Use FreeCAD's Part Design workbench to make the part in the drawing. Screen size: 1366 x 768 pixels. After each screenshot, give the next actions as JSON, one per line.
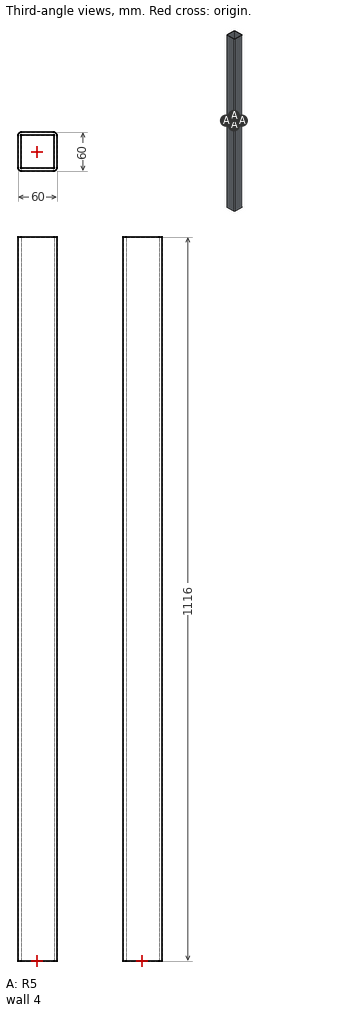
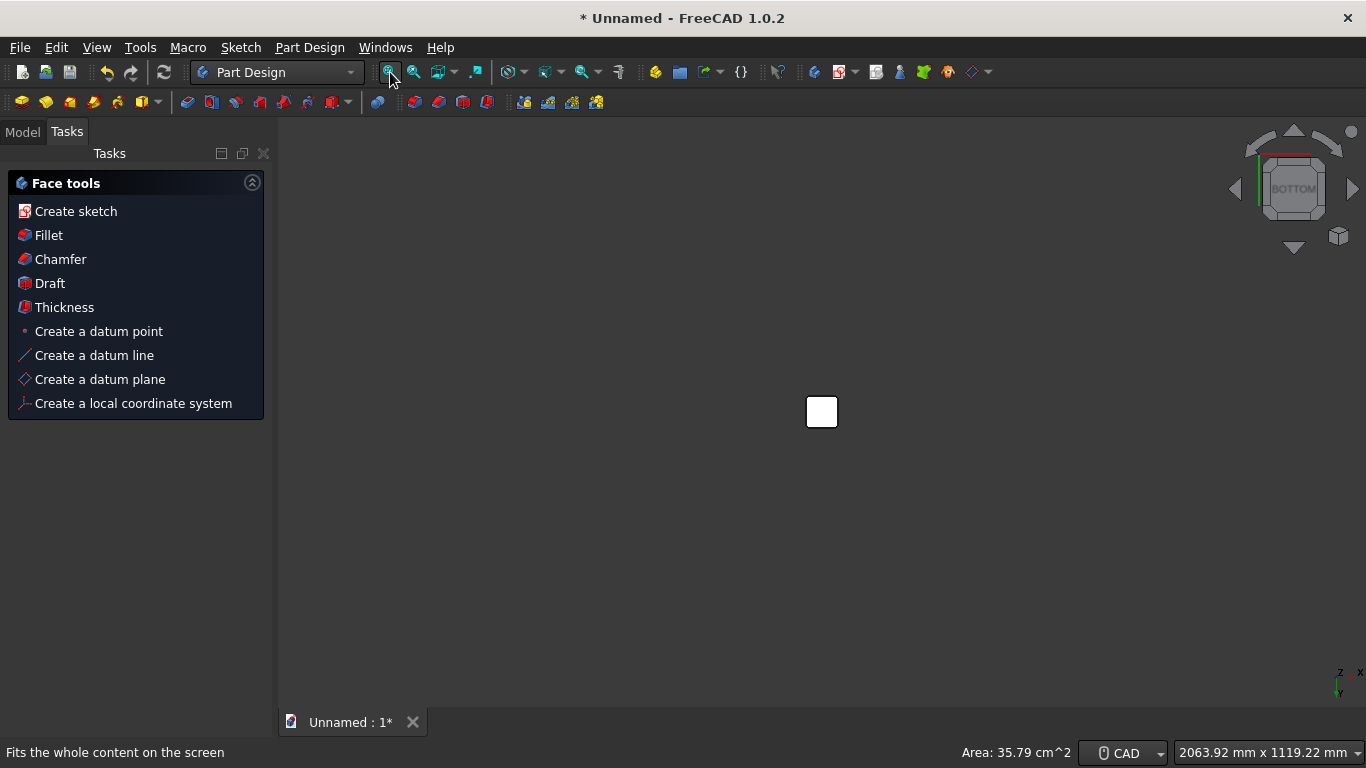
{"action": "left_click", "coordinate": [822, 411], "text": "ctrl"}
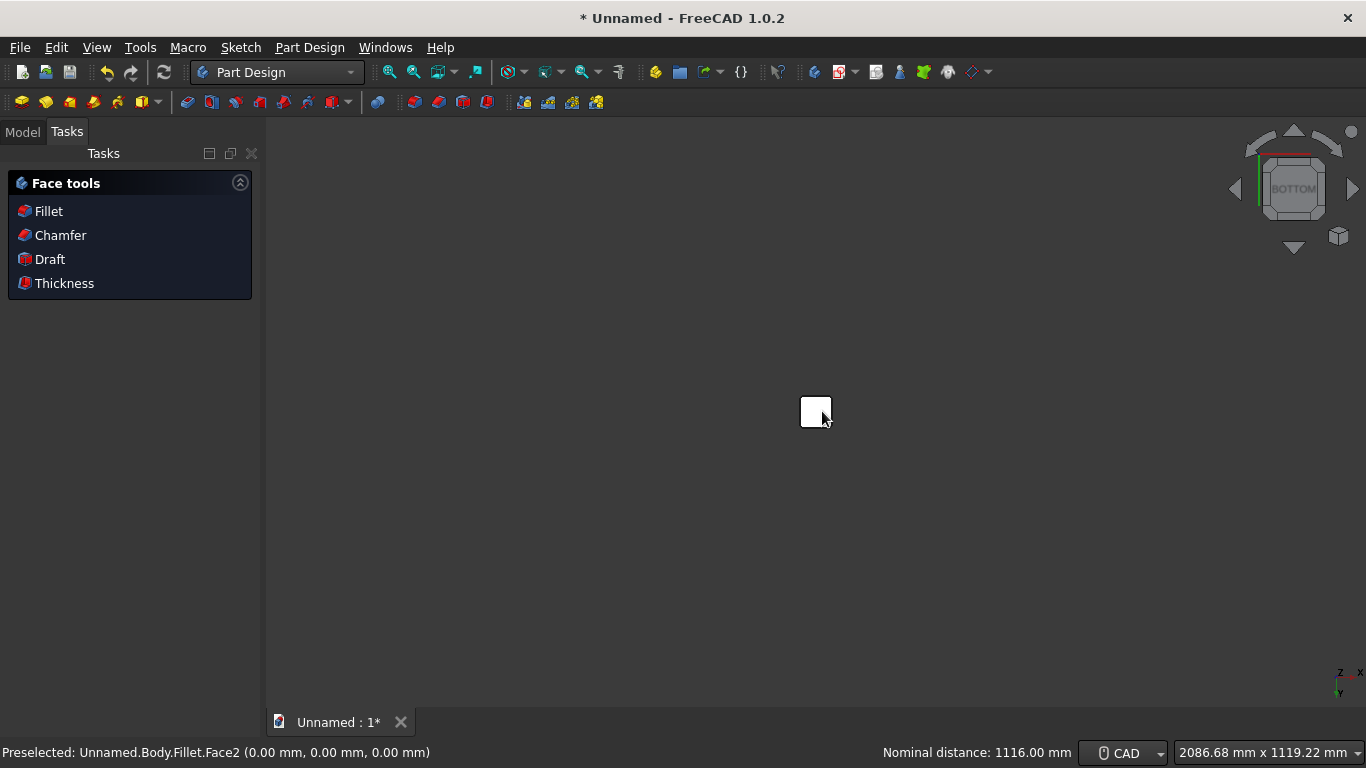
{"action": "left_click", "coordinate": [488, 102]}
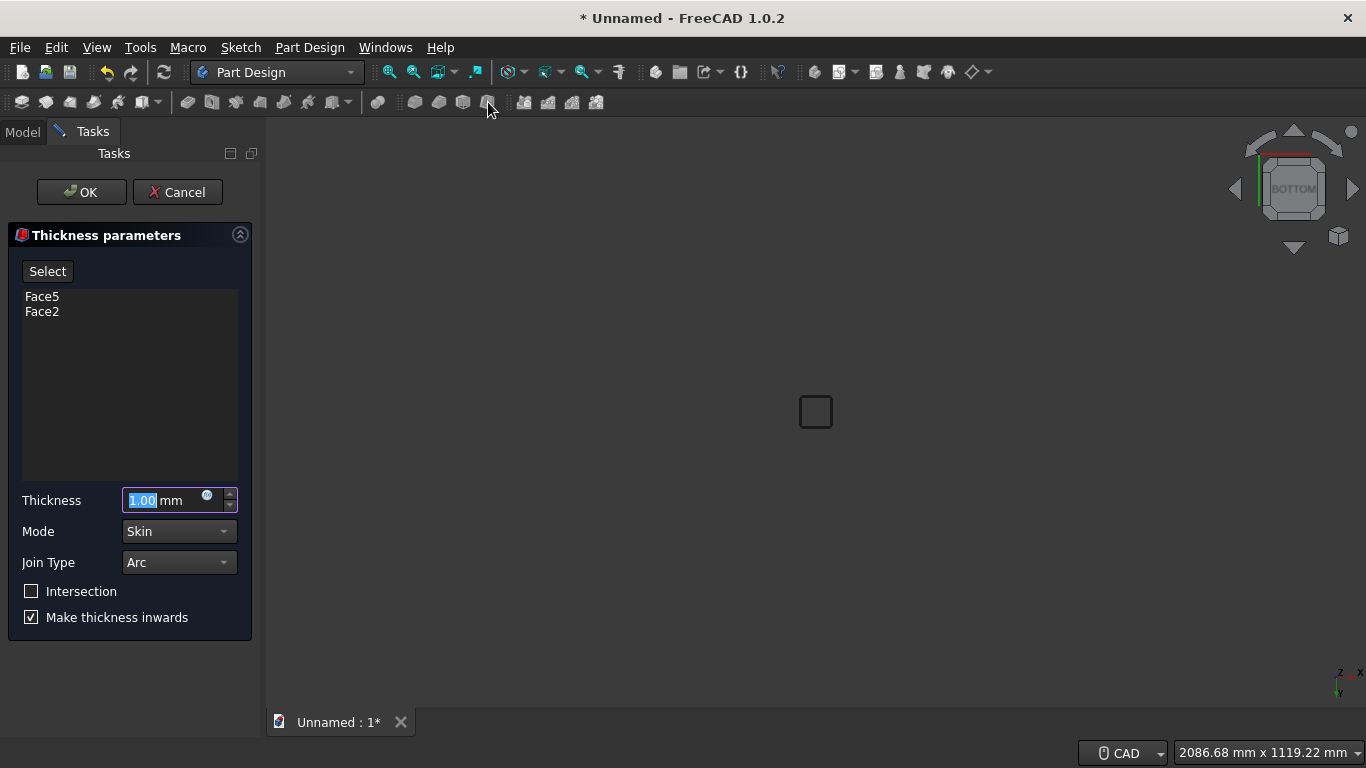
{"action": "type", "text": "4"}
{"action": "key", "text": "Tab"}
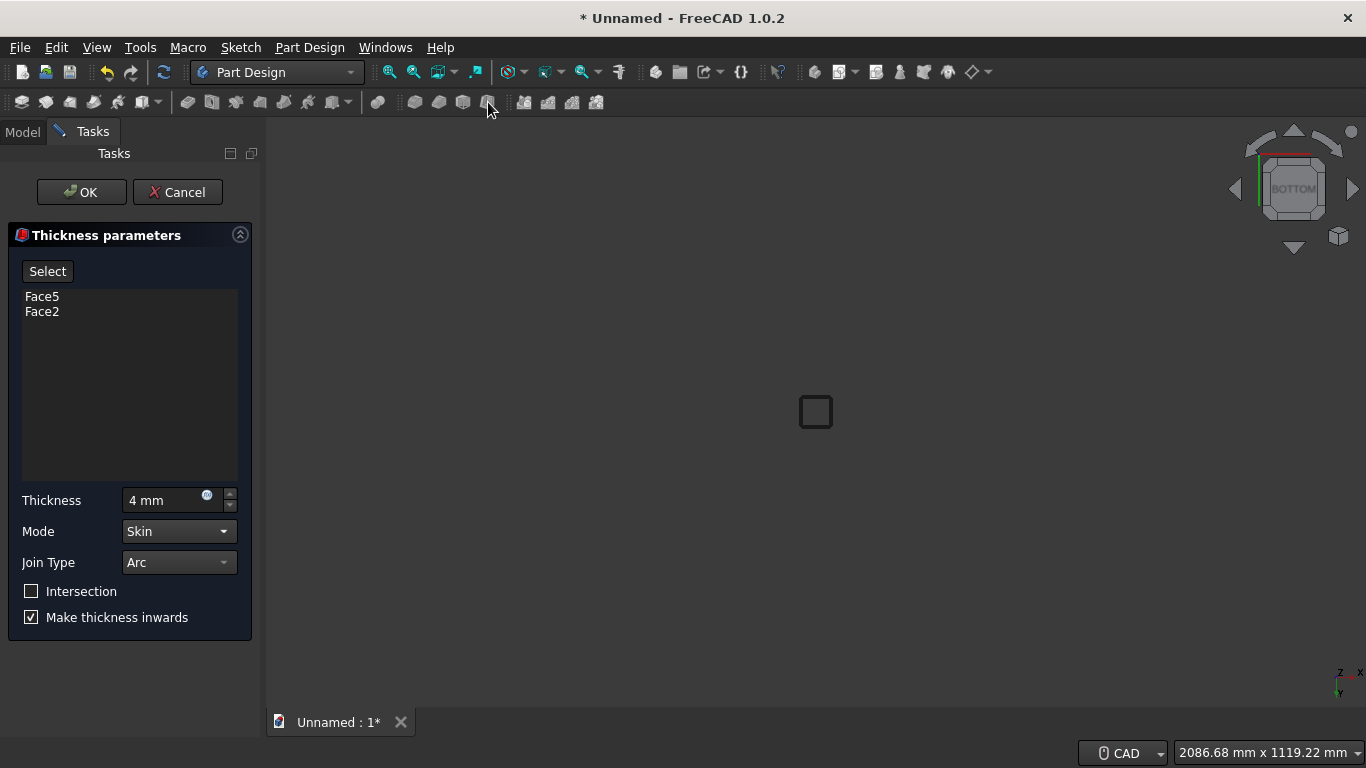
{"action": "left_click", "coordinate": [180, 562]}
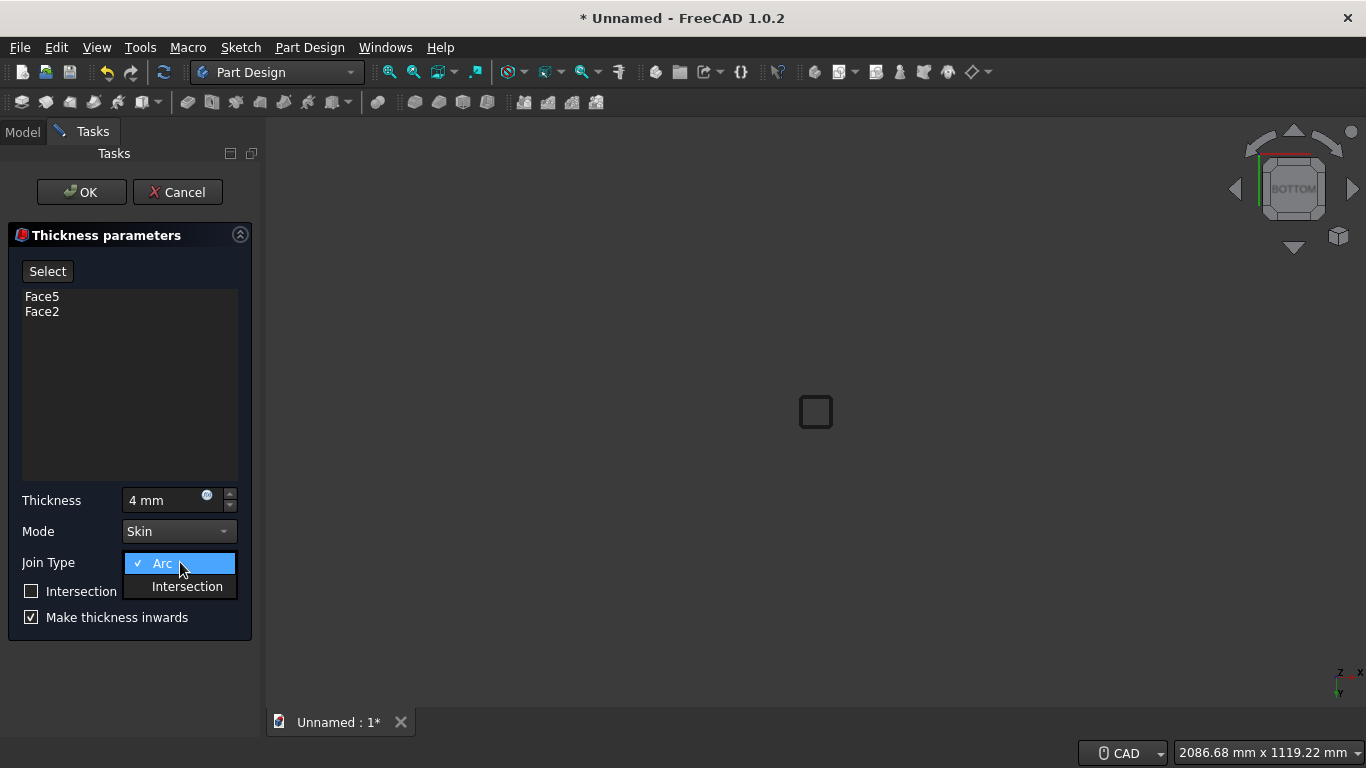
{"action": "left_click", "coordinate": [179, 586]}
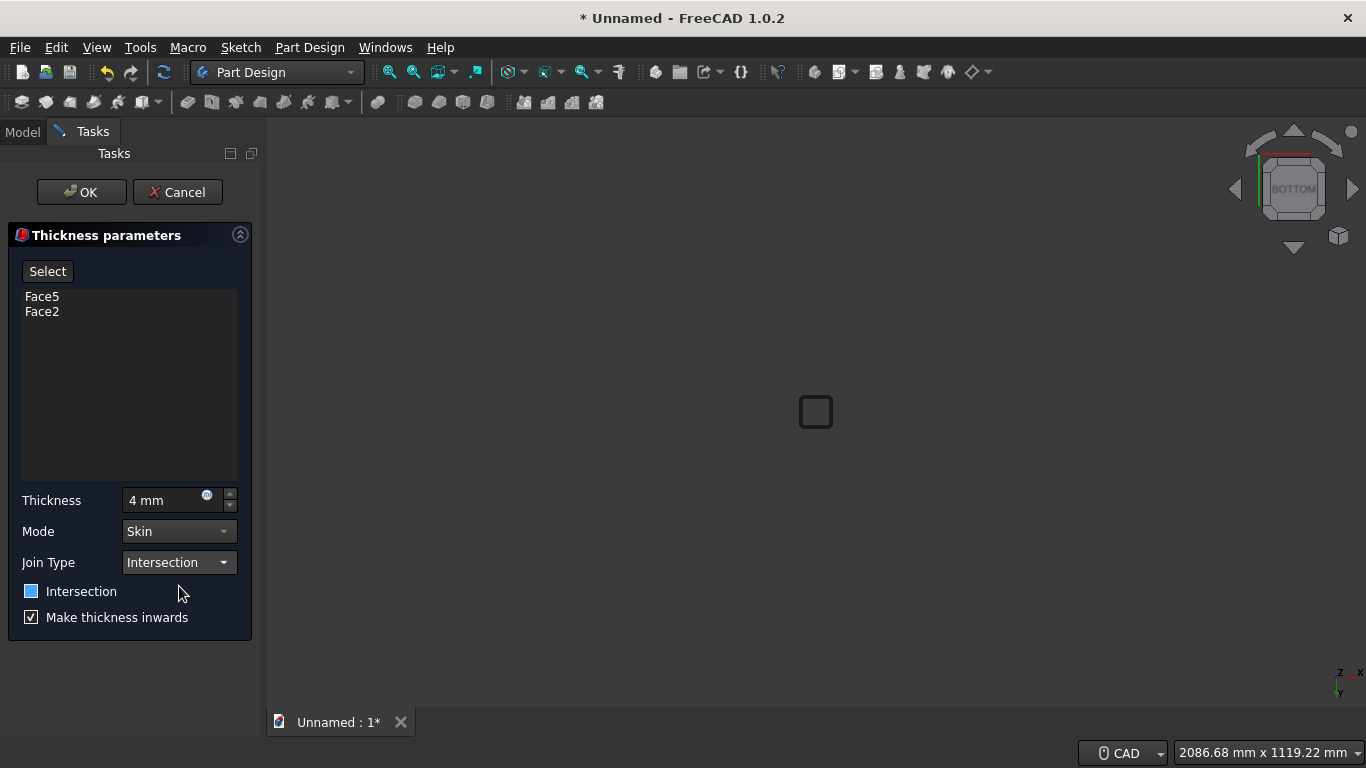
{"action": "left_click", "coordinate": [82, 192]}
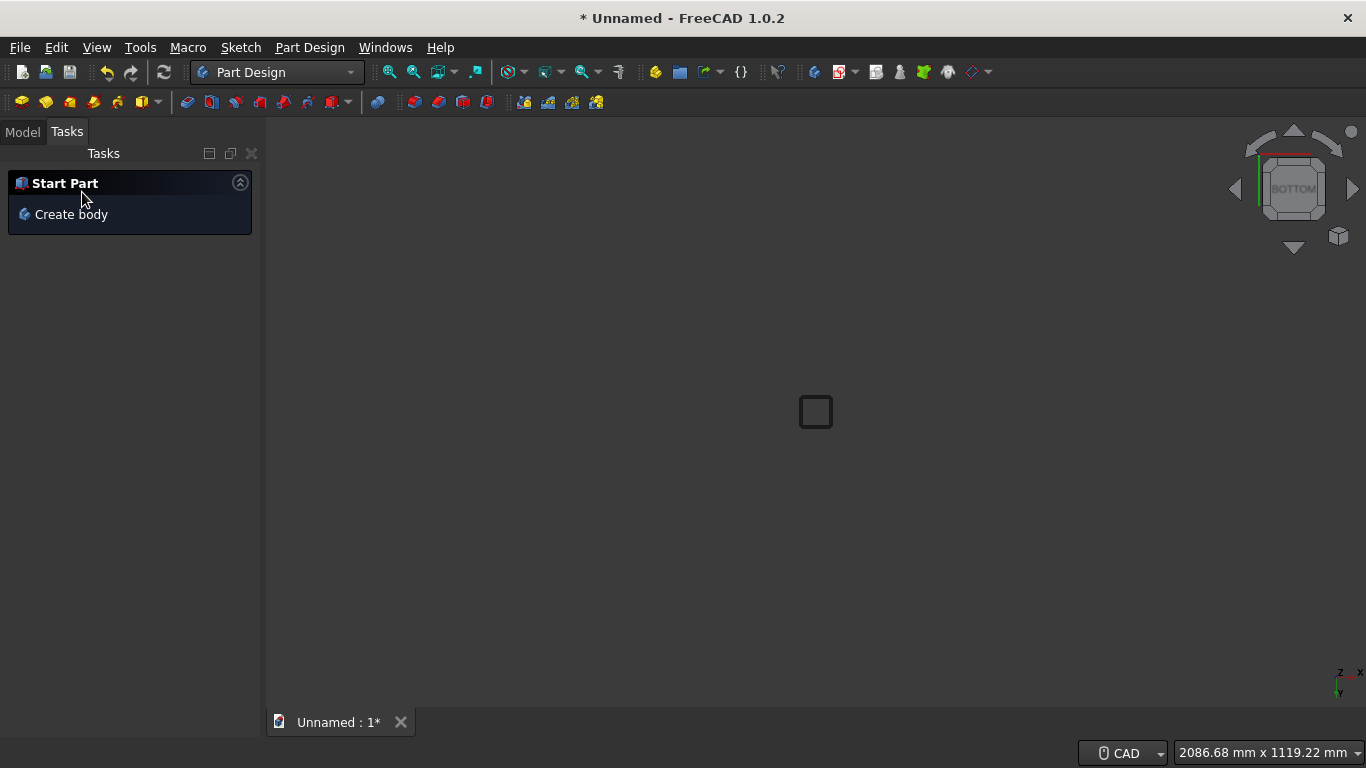
{"action": "key", "text": "0"}